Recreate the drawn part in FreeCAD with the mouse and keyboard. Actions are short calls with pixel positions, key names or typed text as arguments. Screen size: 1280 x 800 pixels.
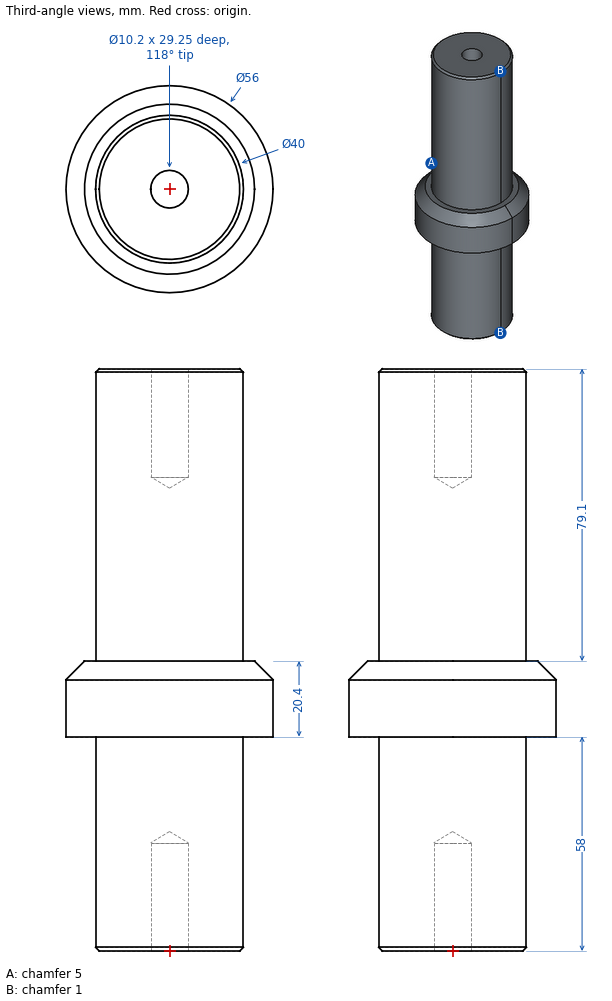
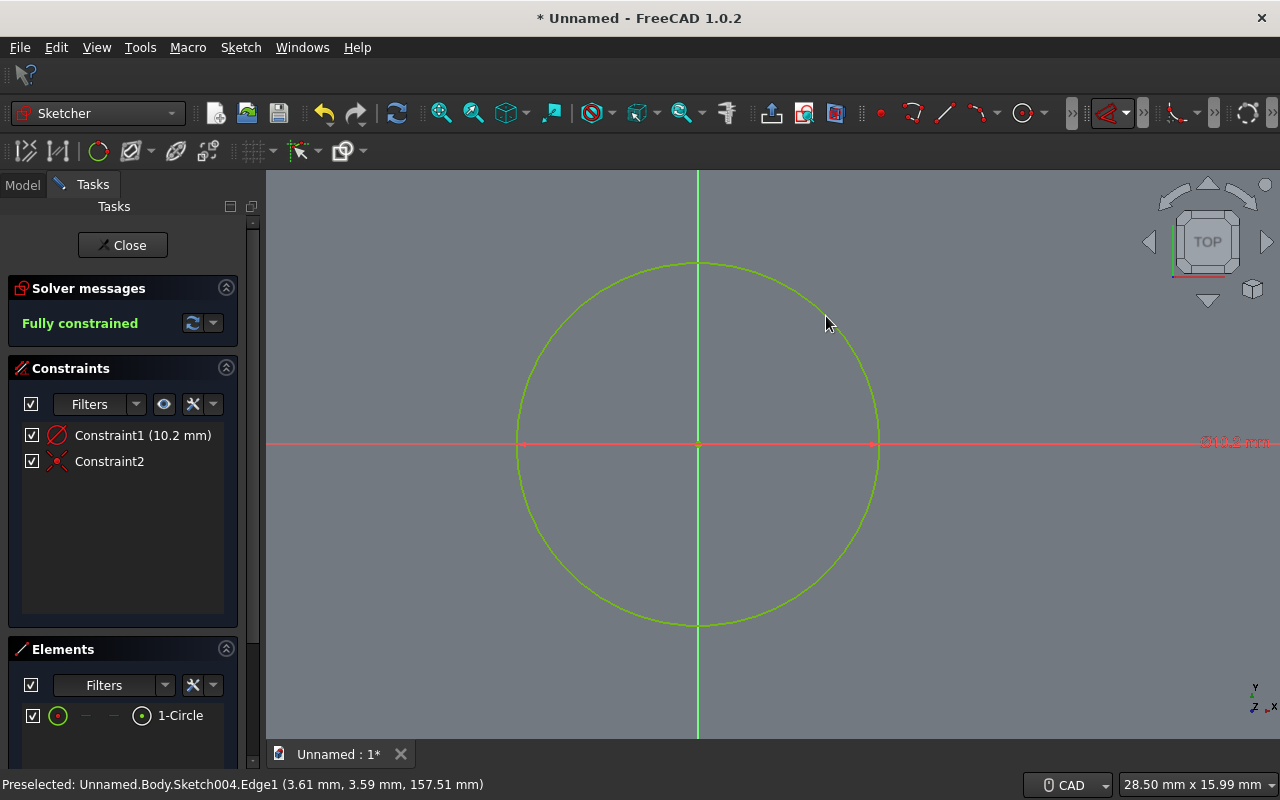
click(123, 245)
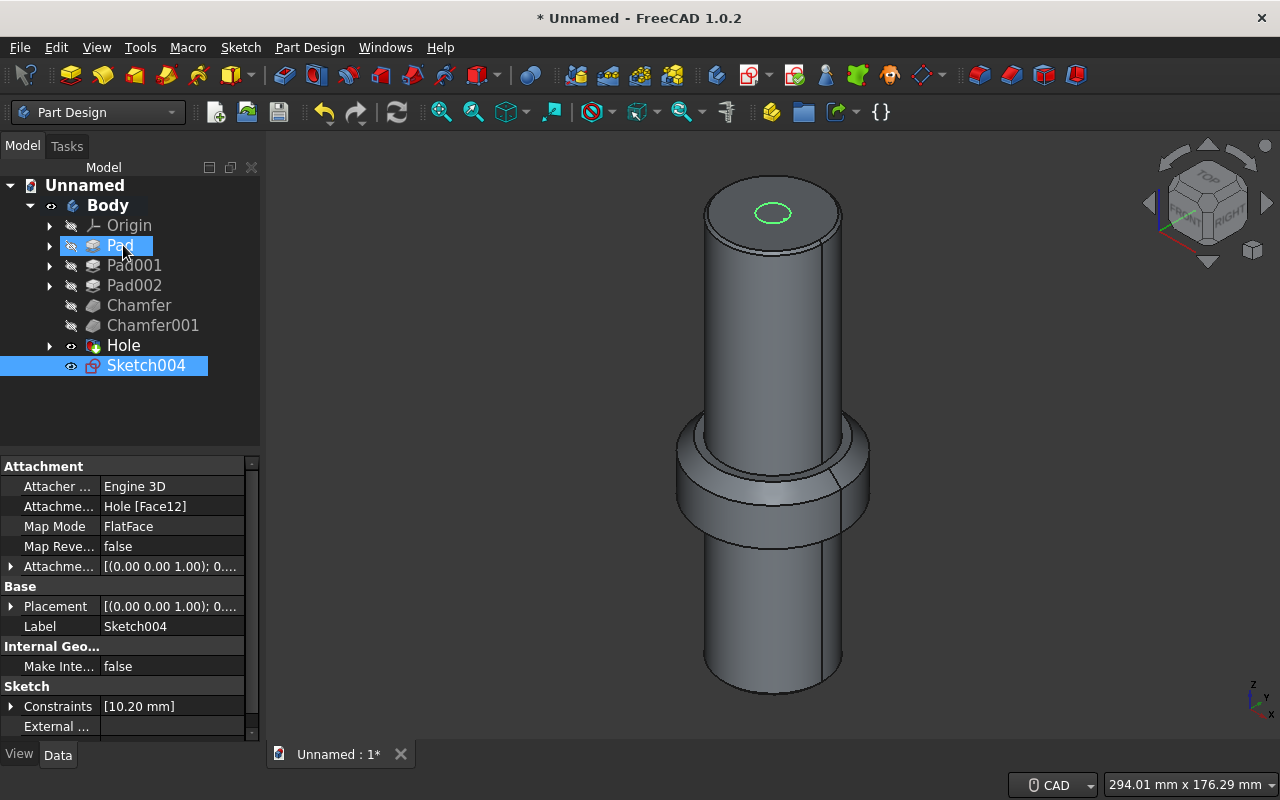
click(318, 76)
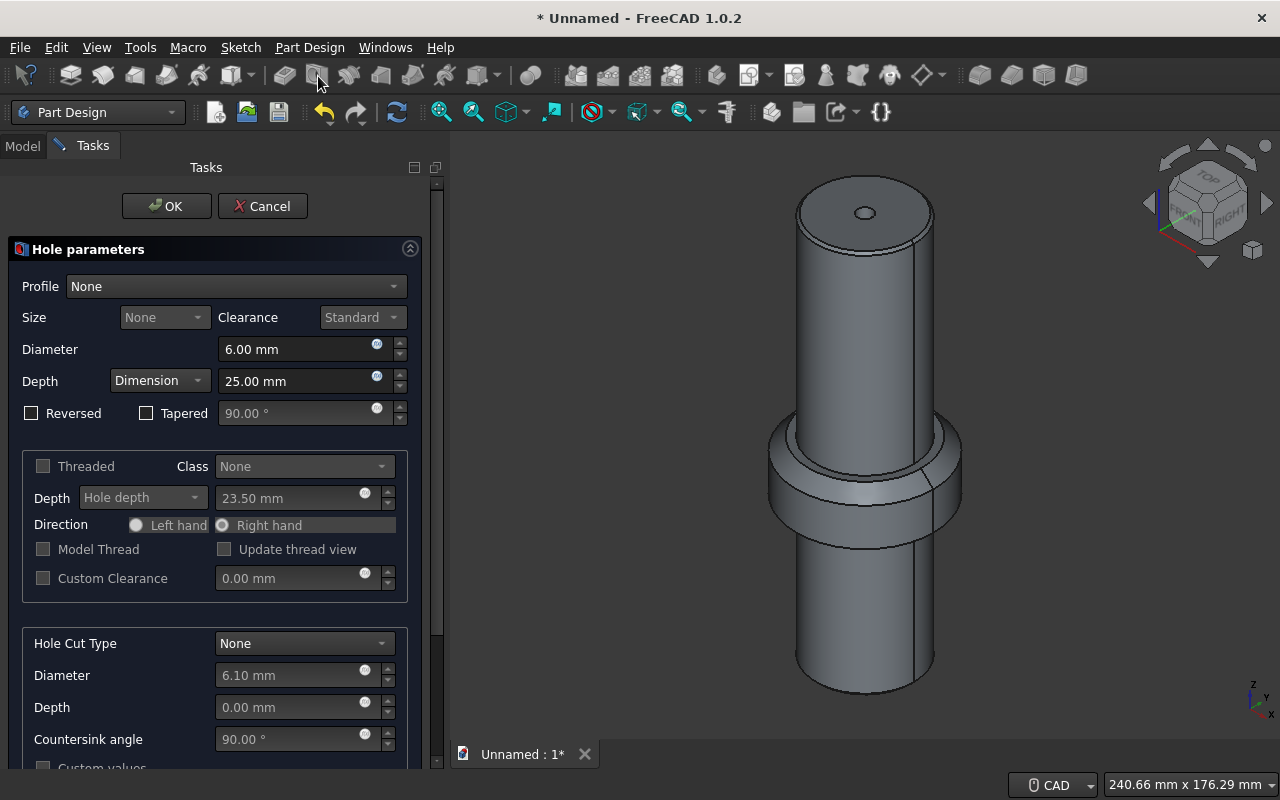
triple_click(305, 349)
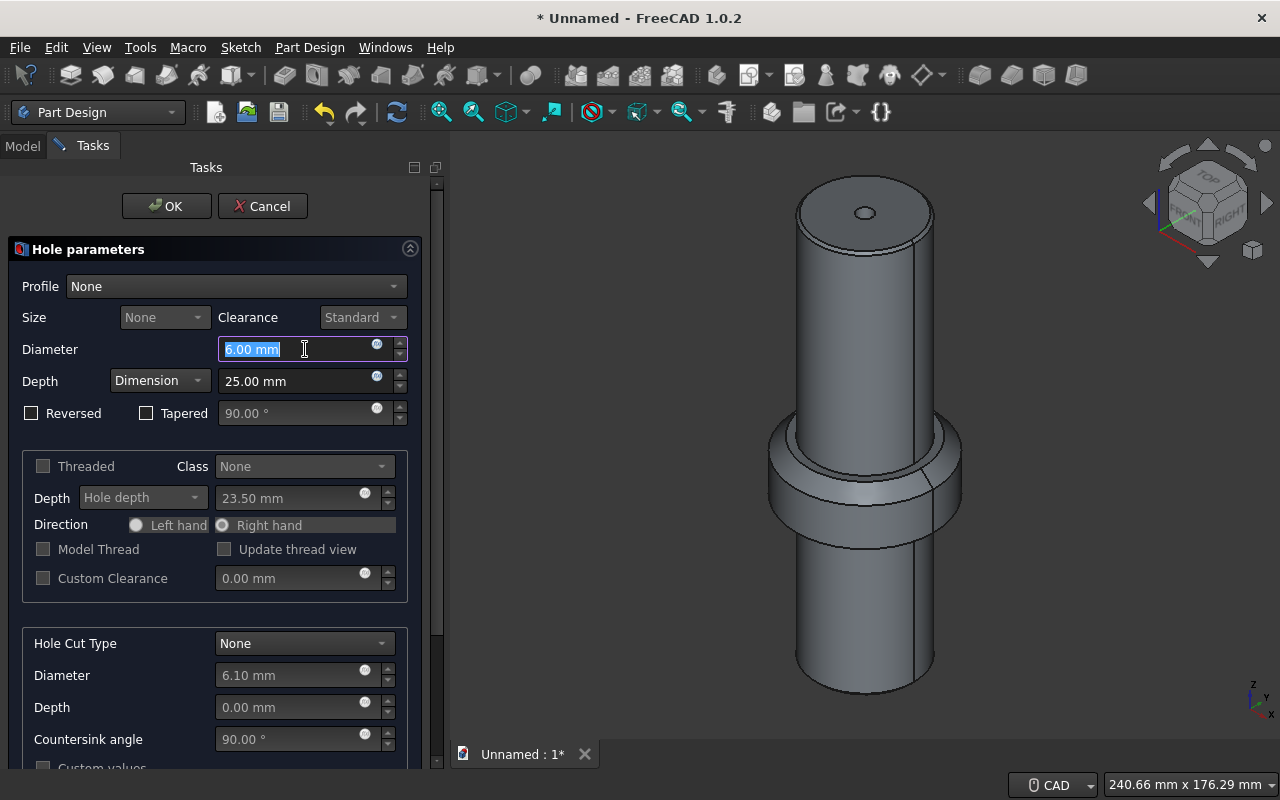
text(10.2)
key(Tab)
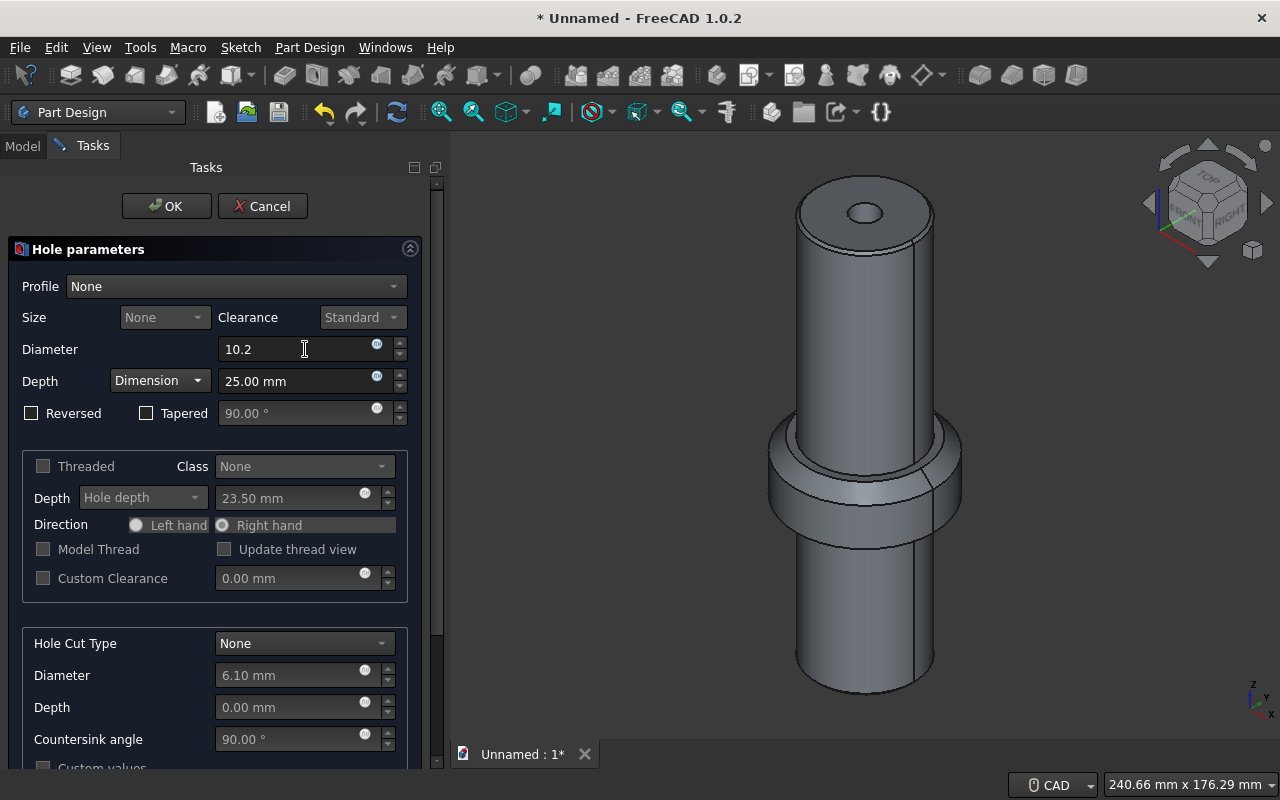
triple_click(305, 381)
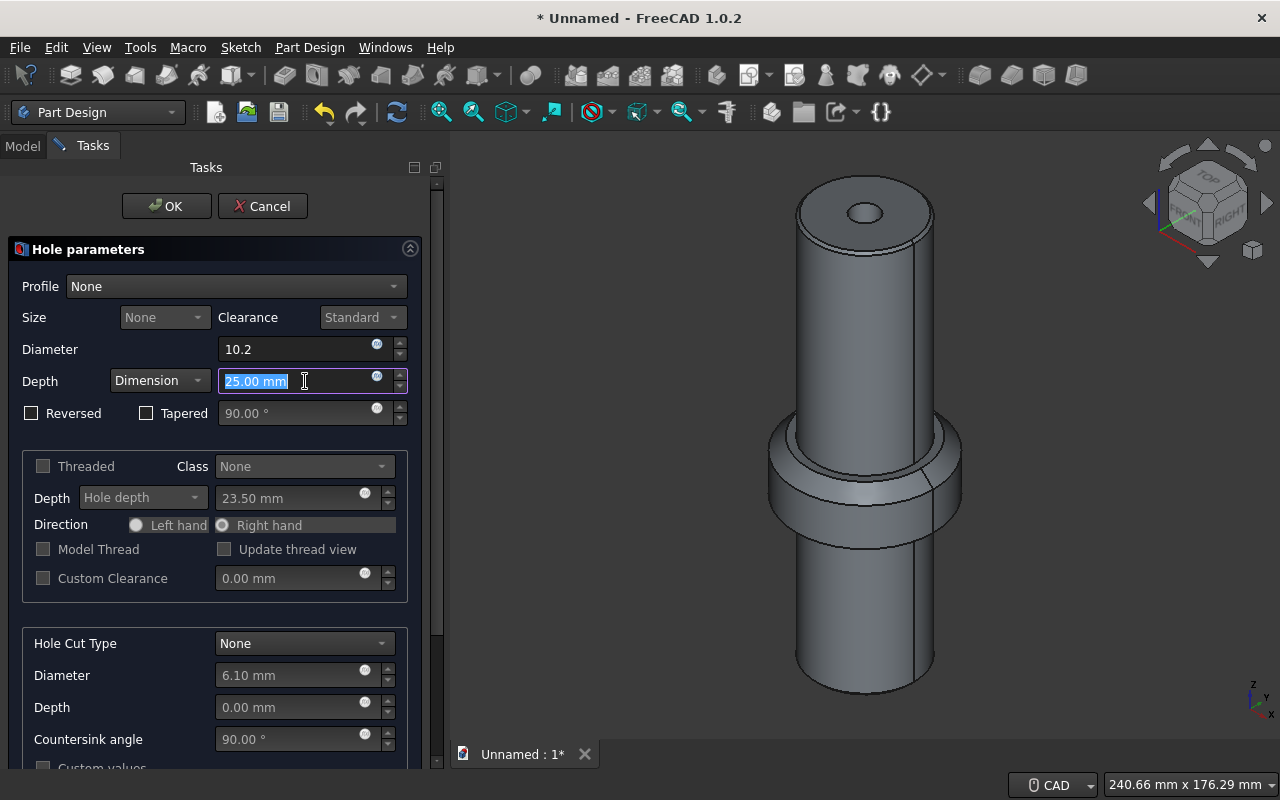
text(29.25)
key(Tab)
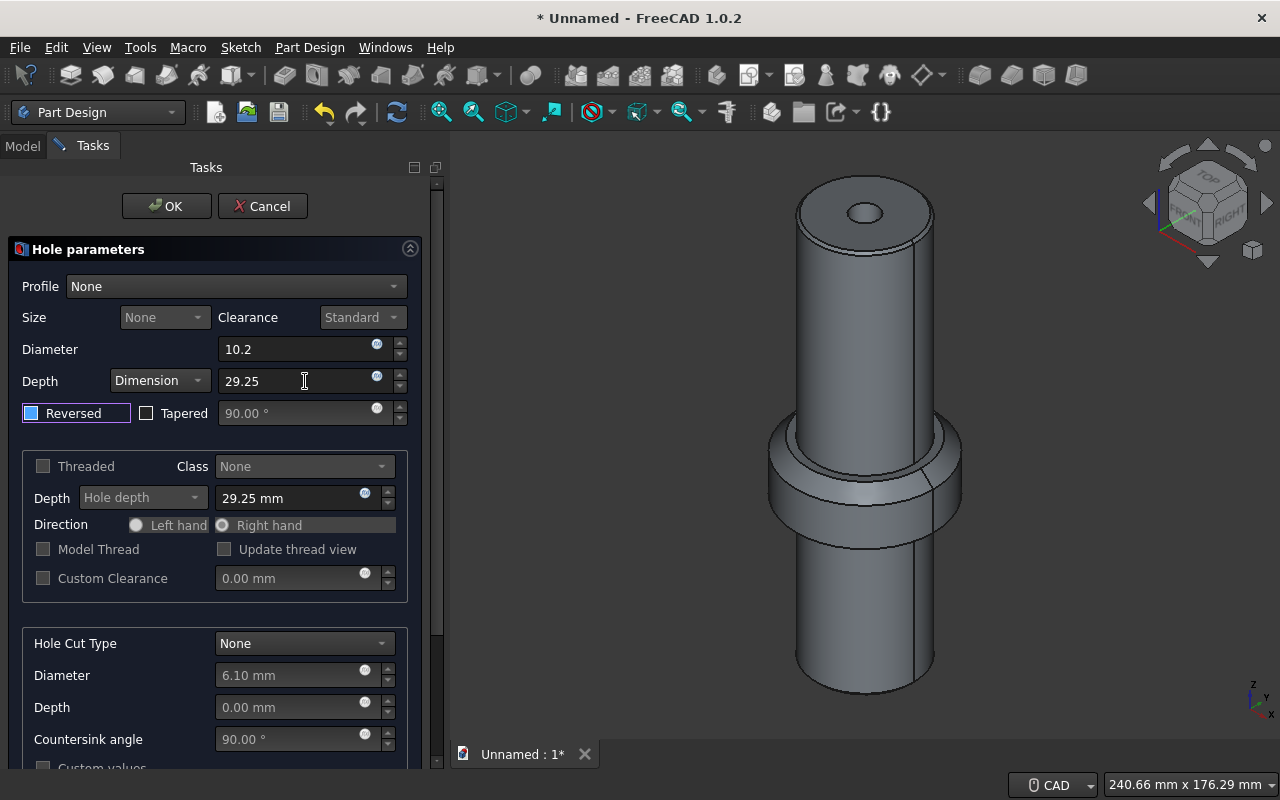
click(167, 206)